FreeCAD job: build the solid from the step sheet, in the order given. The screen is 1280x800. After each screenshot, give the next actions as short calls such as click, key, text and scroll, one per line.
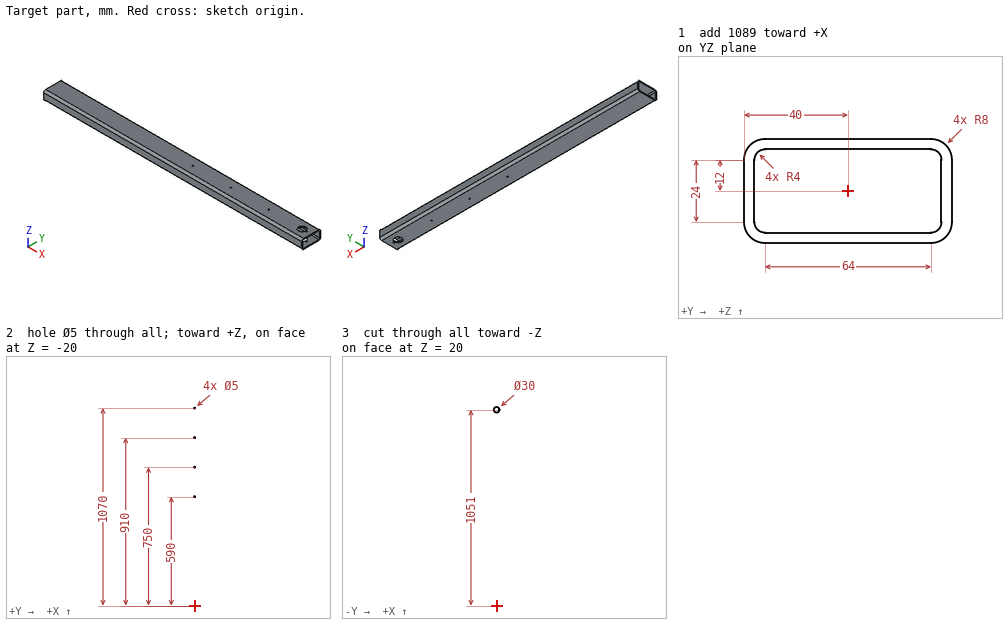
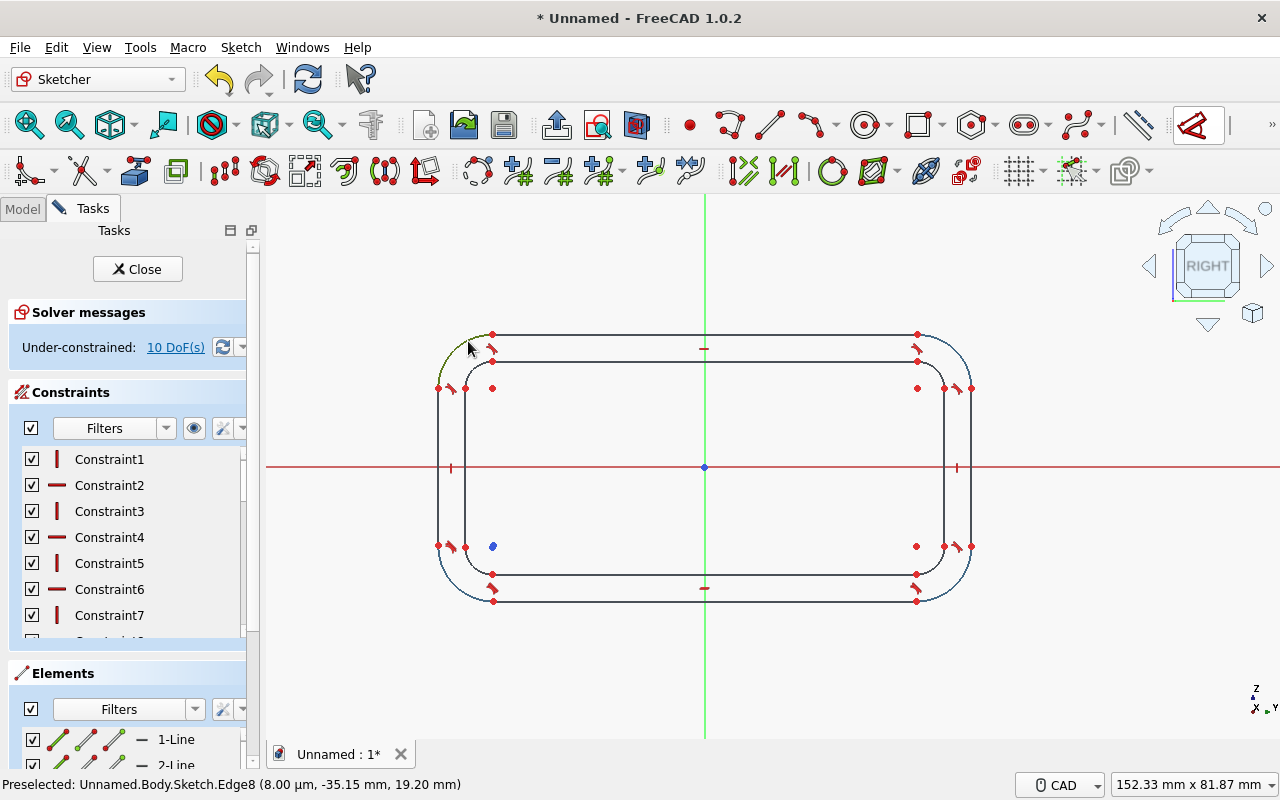
key(e)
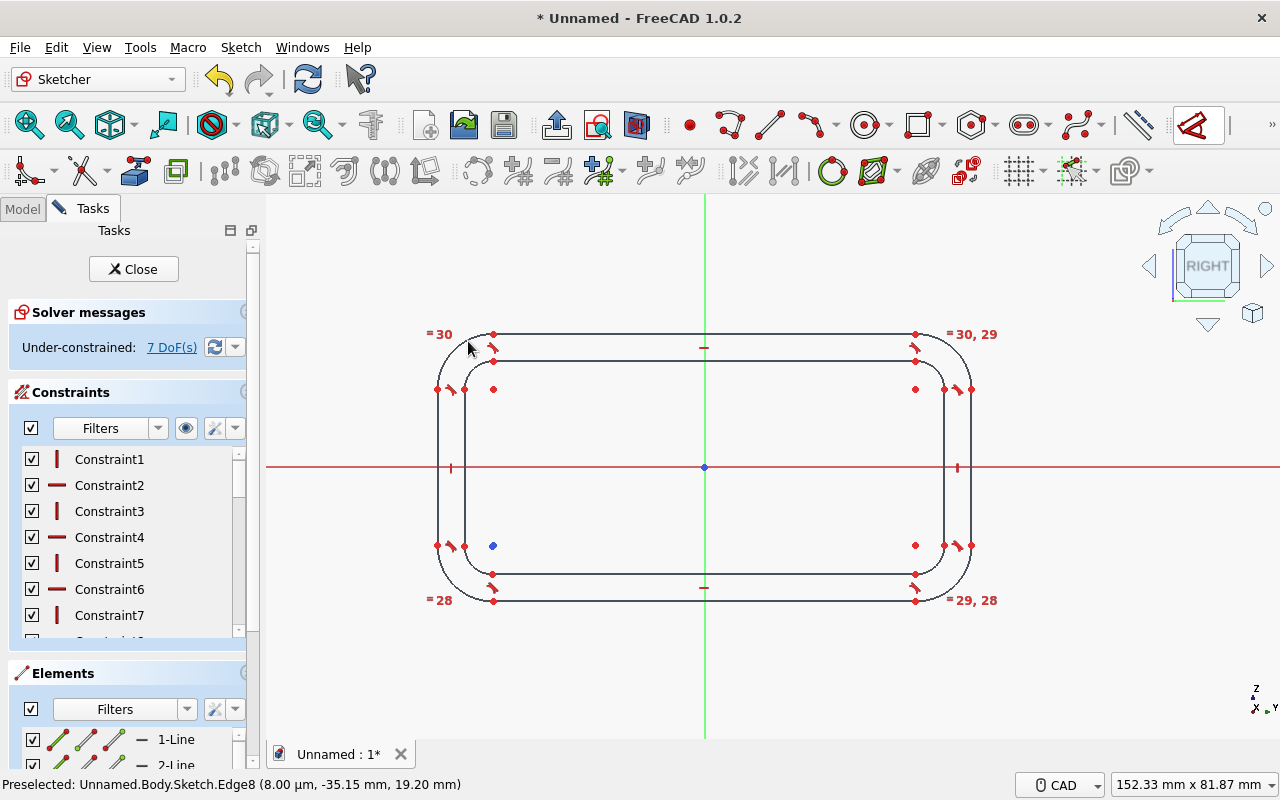
click(480, 364)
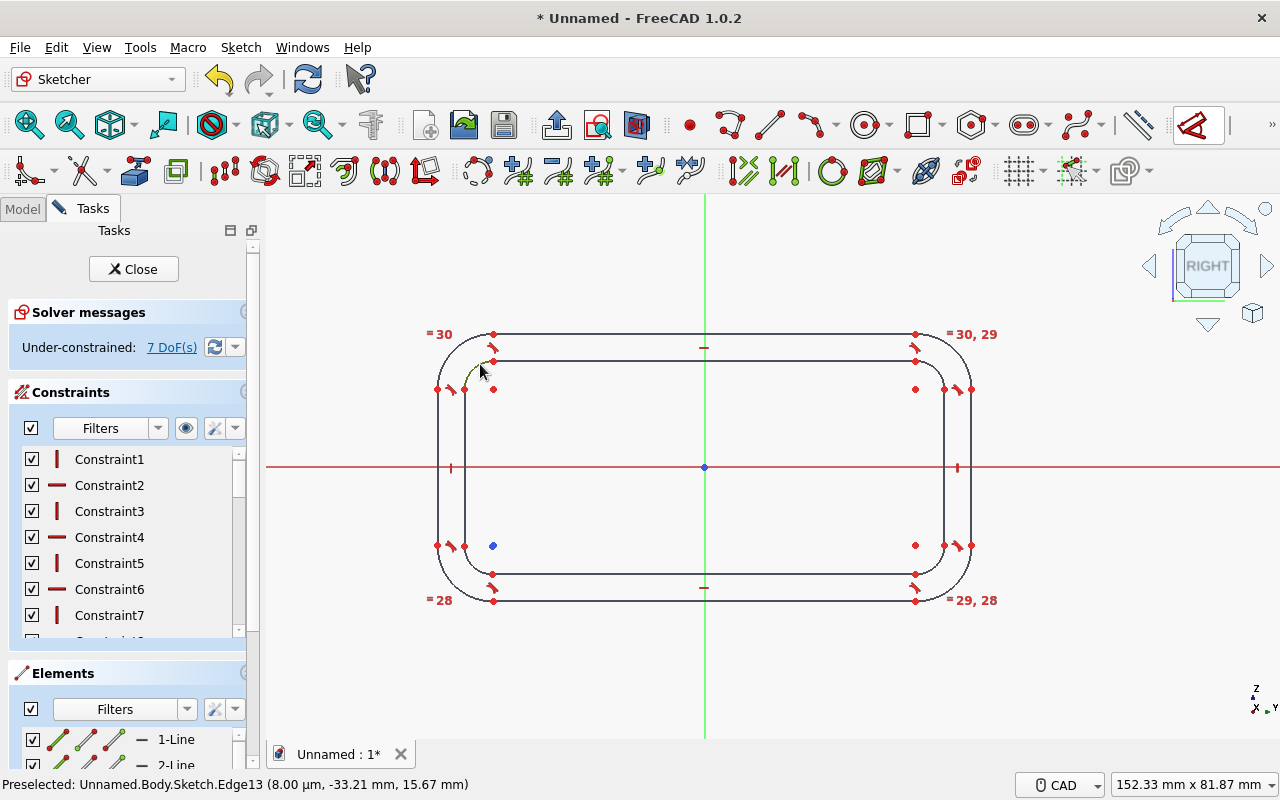
click(468, 559)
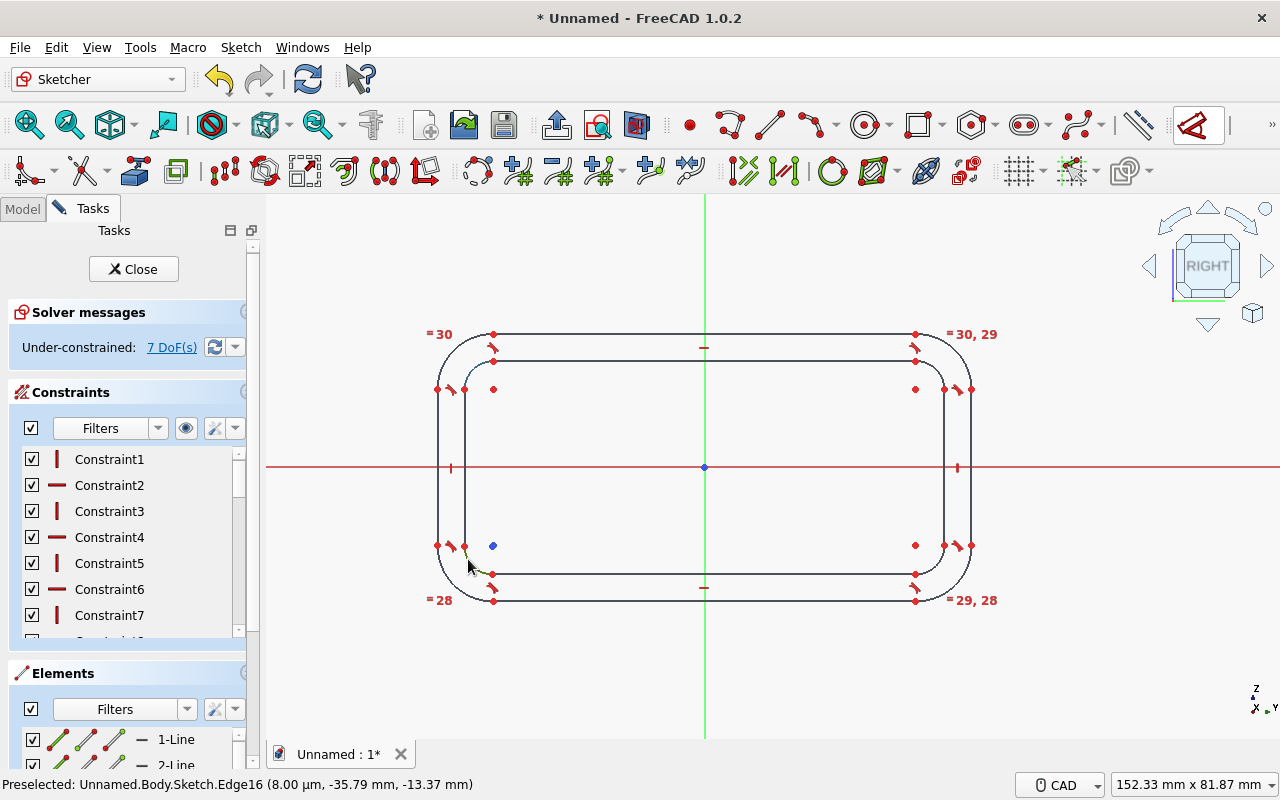
key(e)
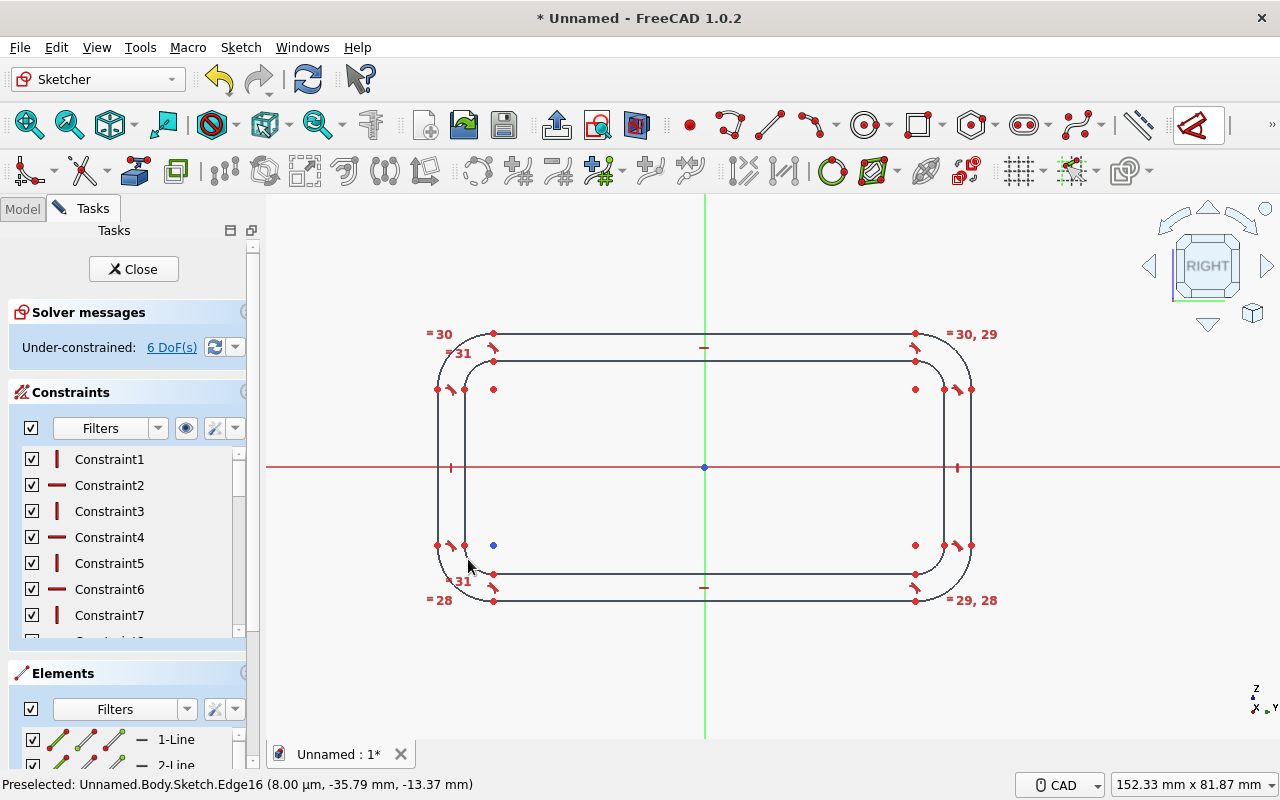
click(1192, 126)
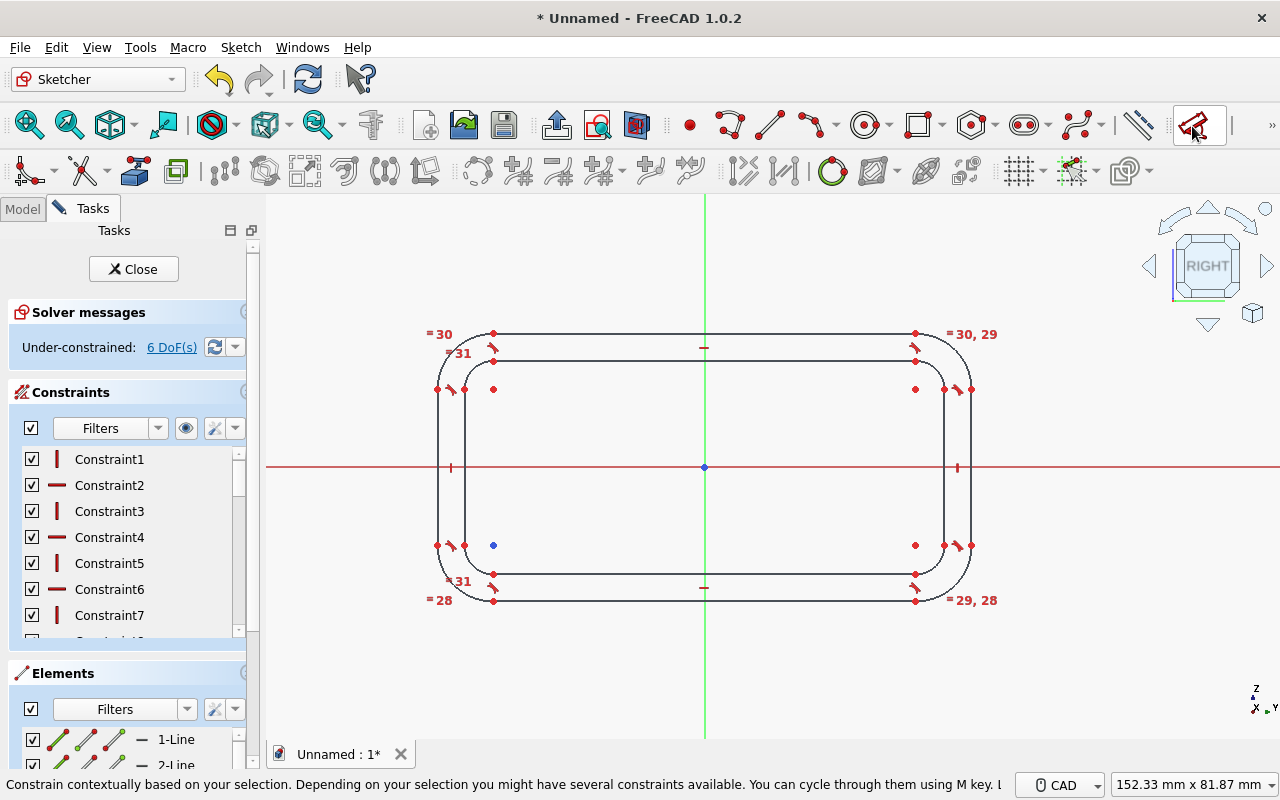
click(444, 571)
click(415, 586)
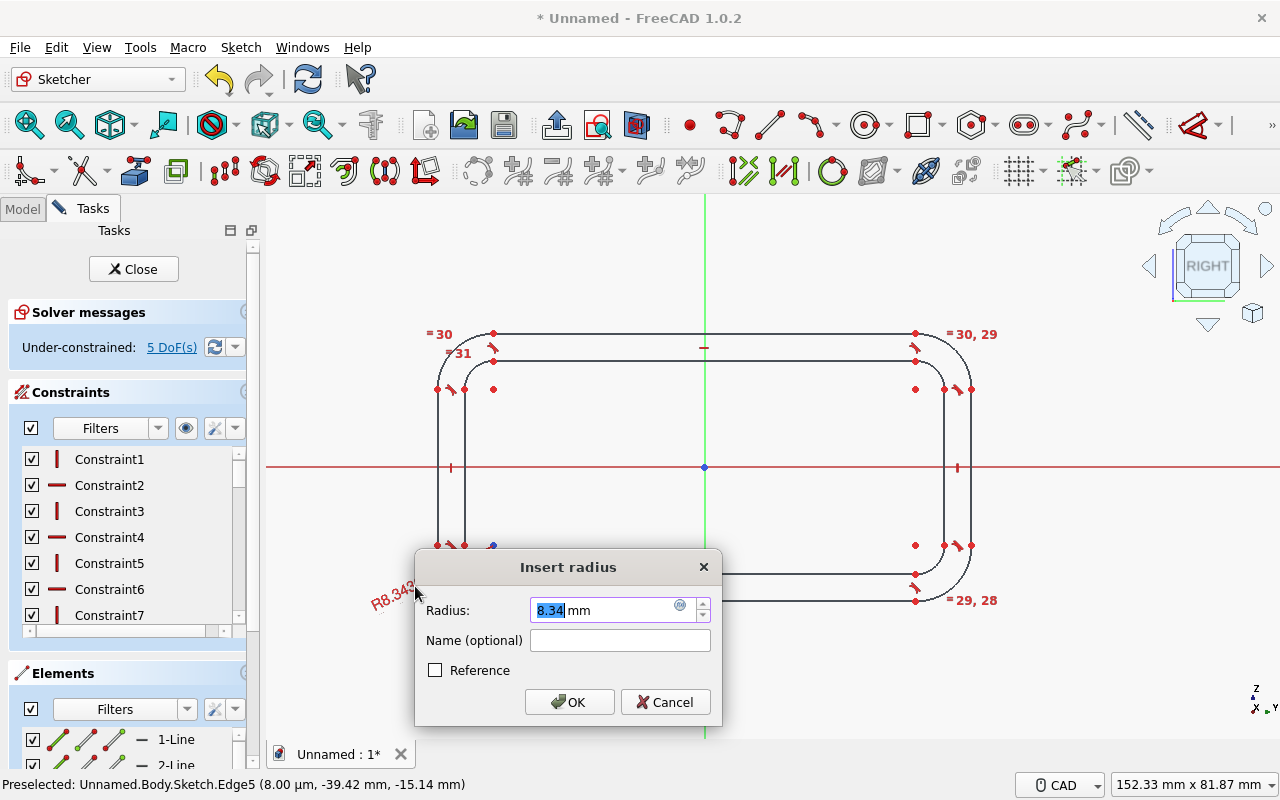
text(8)
key(Return)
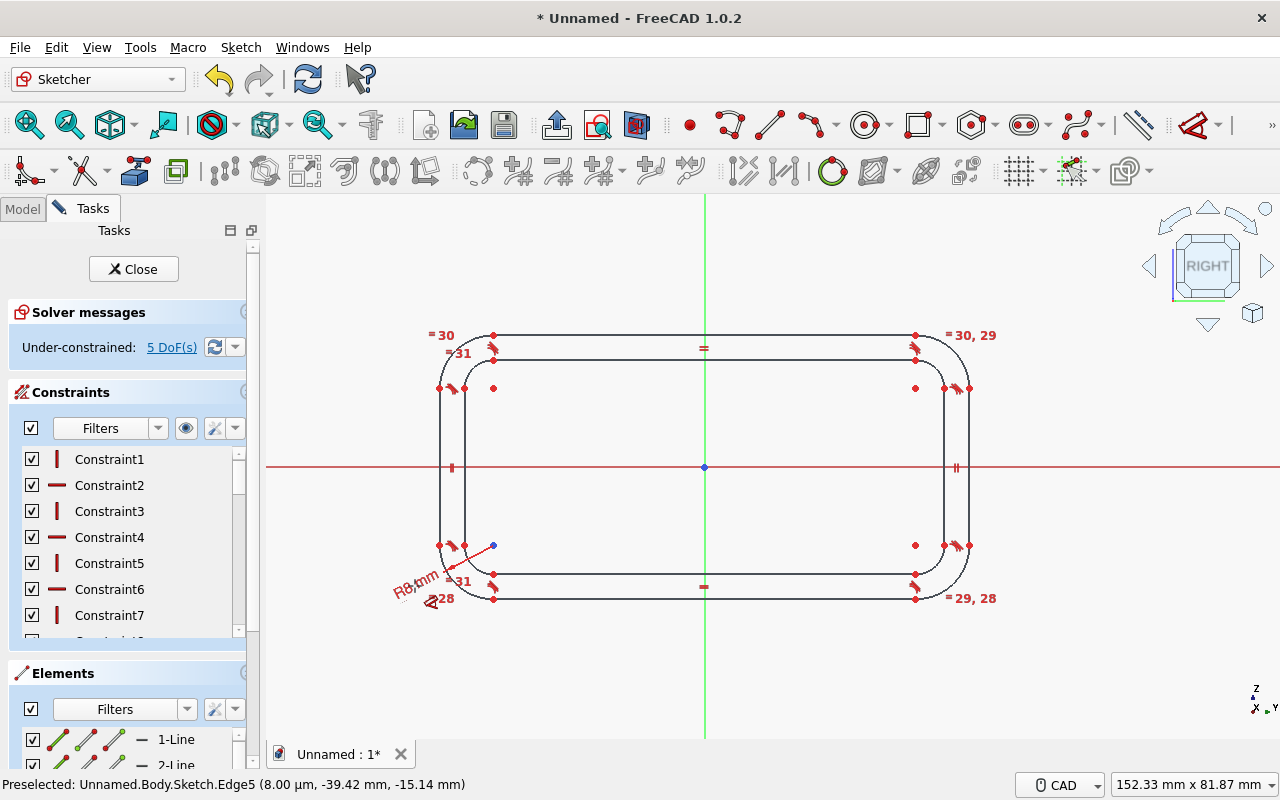
scroll(480, 363, up, 2)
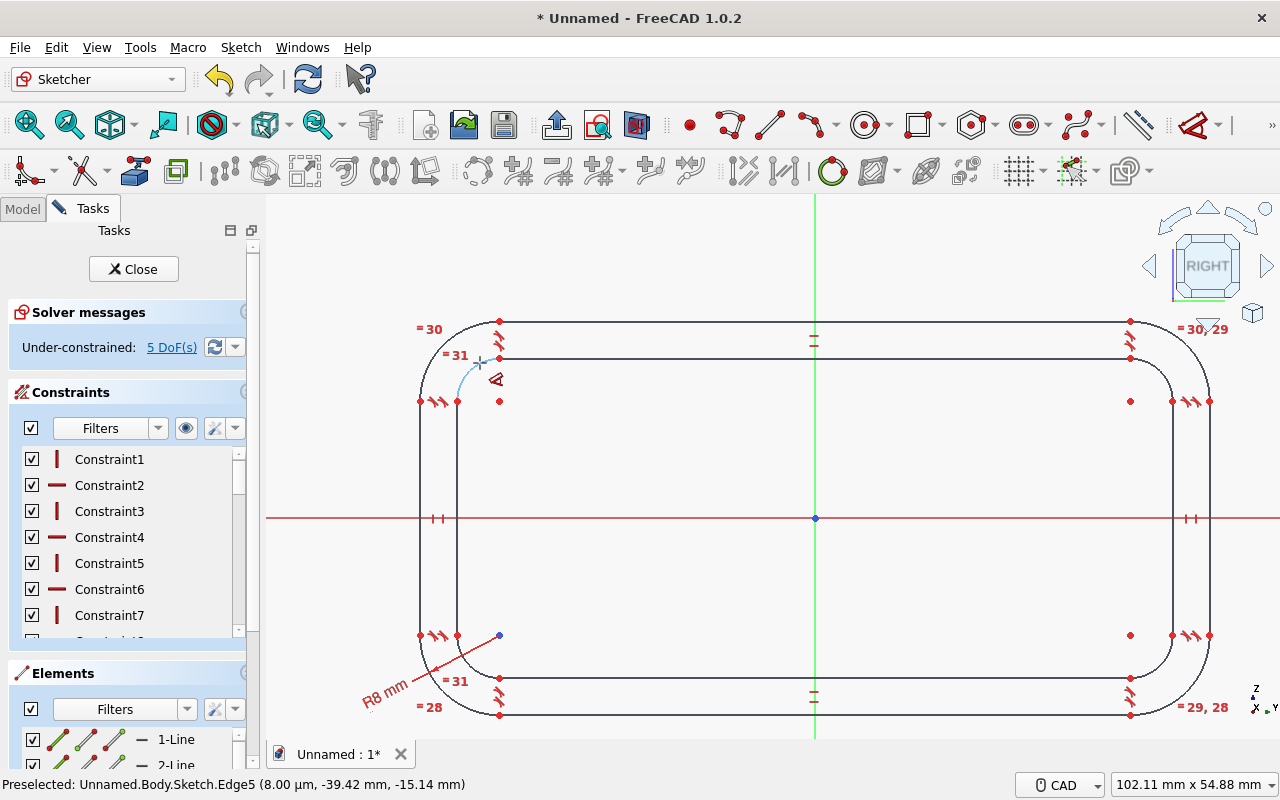
click(480, 363)
click(537, 336)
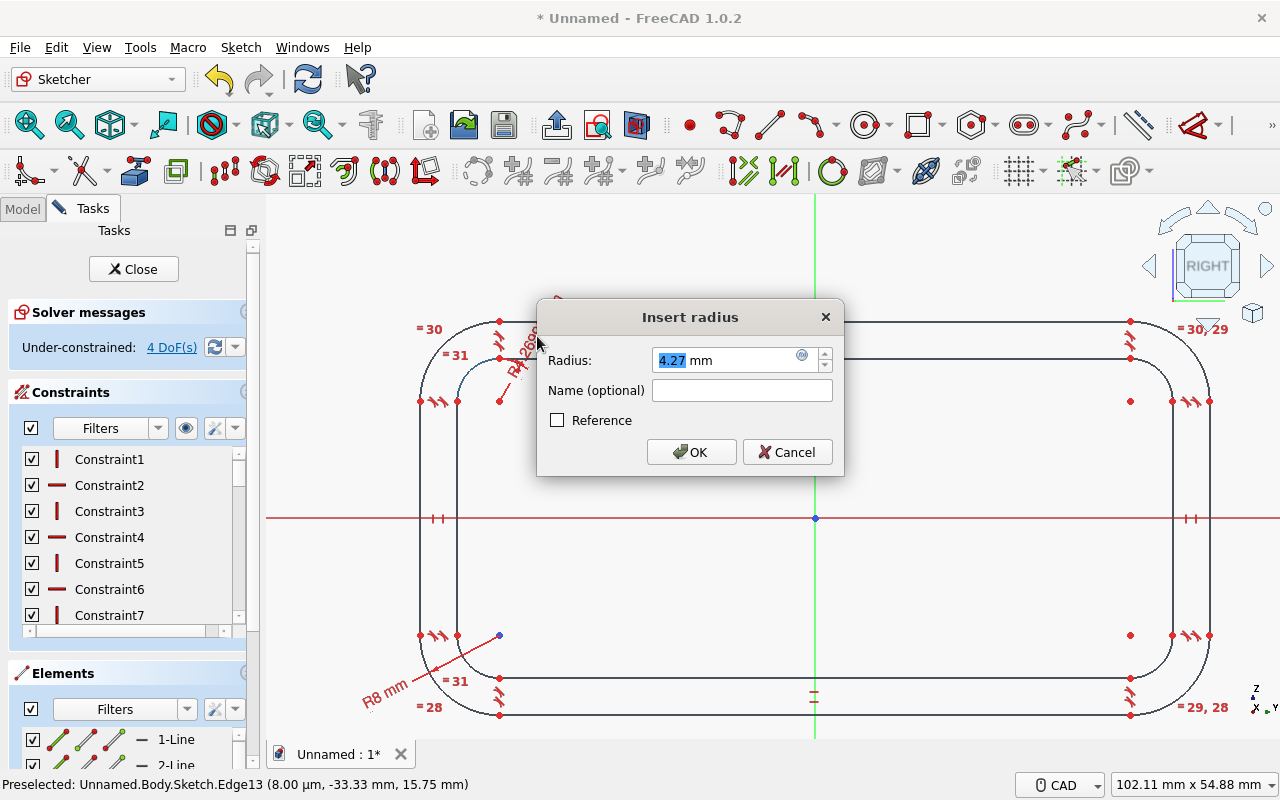
text(4)
key(Return)